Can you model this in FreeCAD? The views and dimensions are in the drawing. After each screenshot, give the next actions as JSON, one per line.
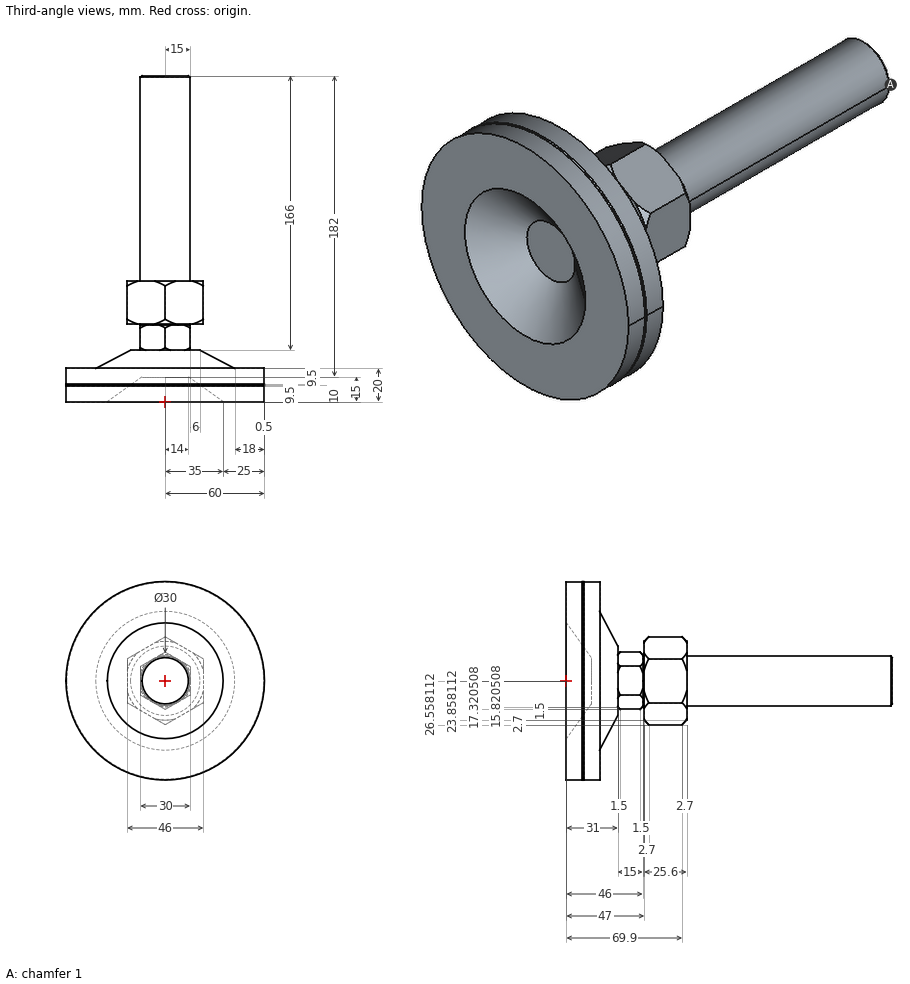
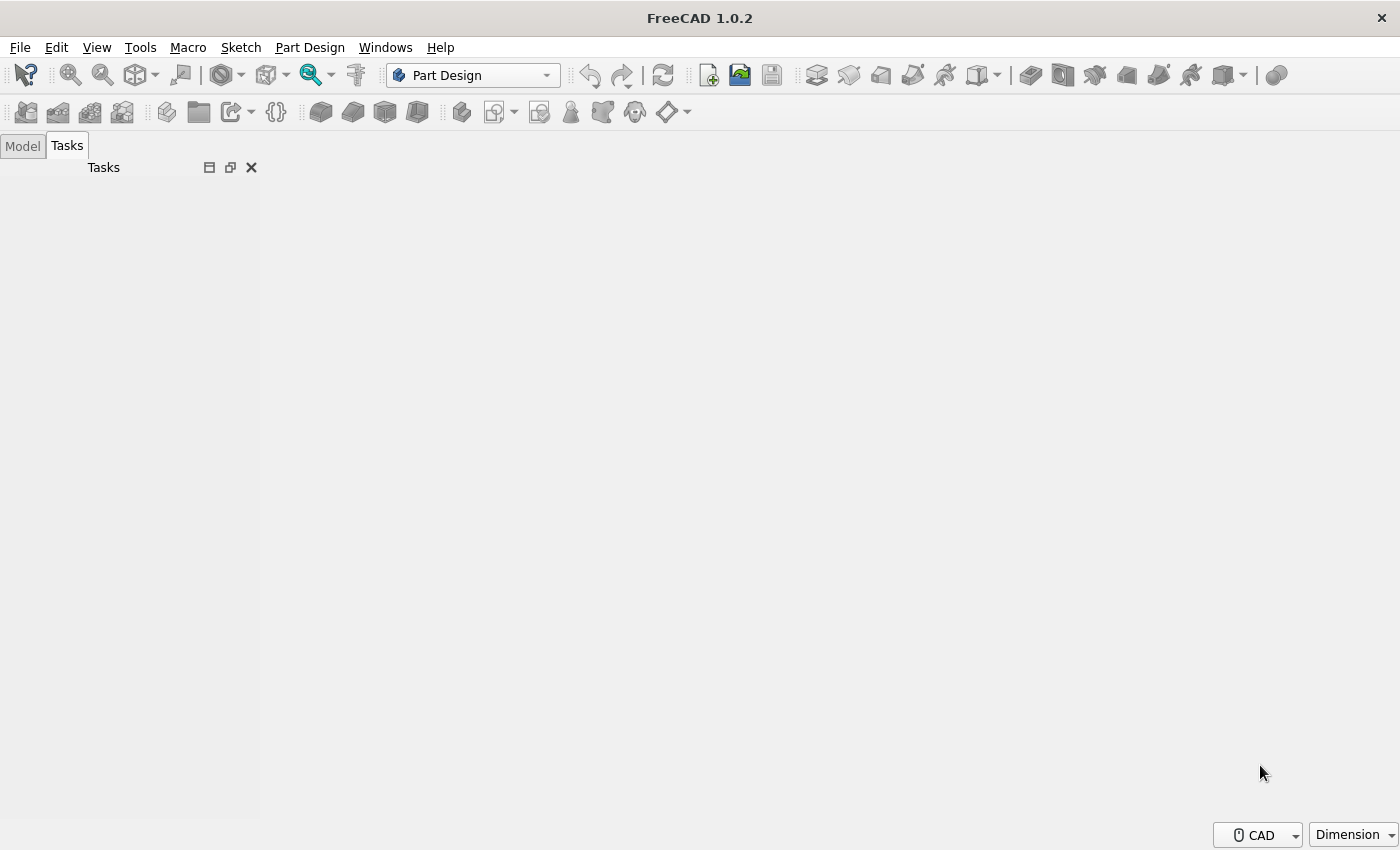
{"action": "key", "text": "ctrl+n"}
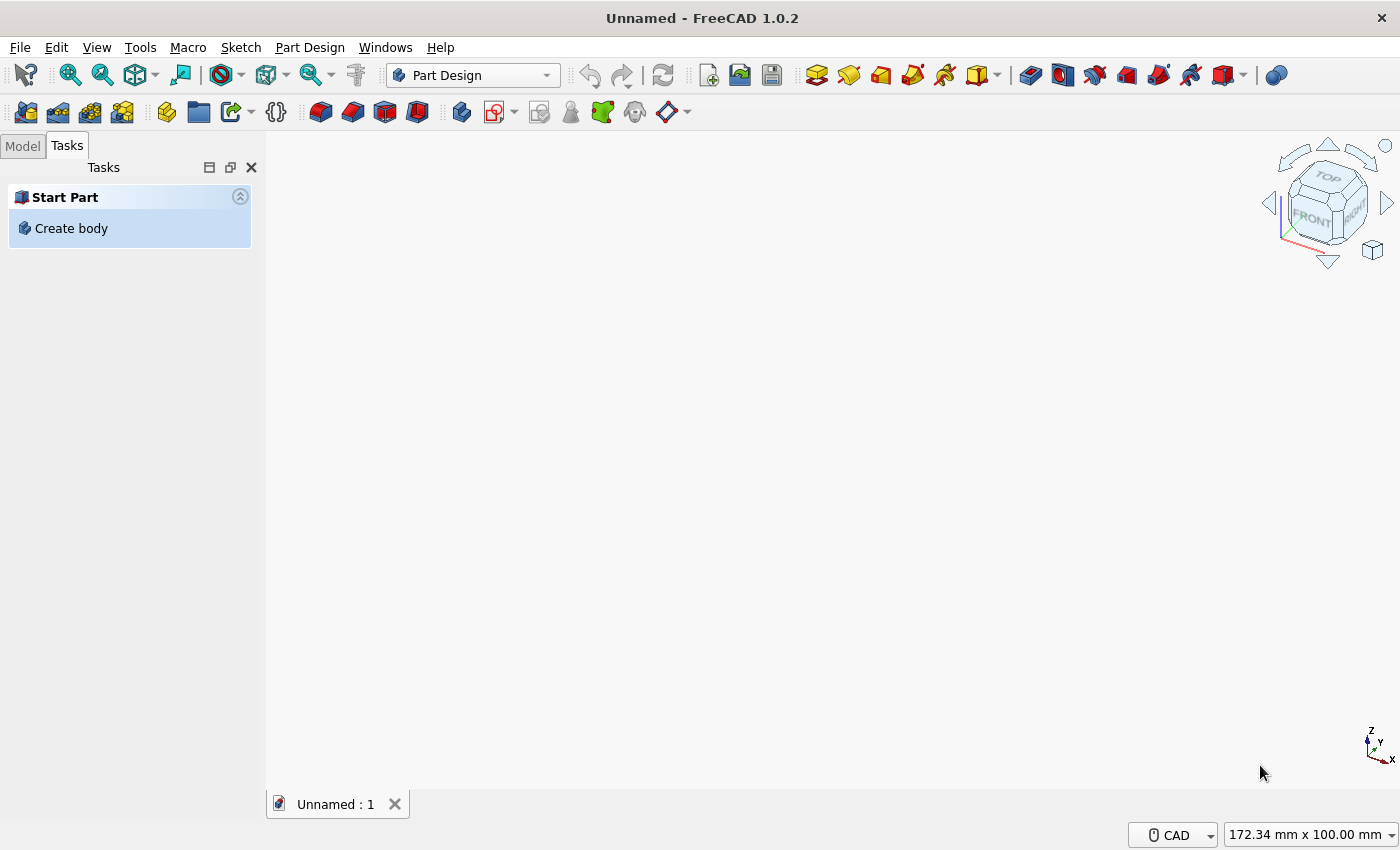
{"action": "left_click", "coordinate": [494, 112]}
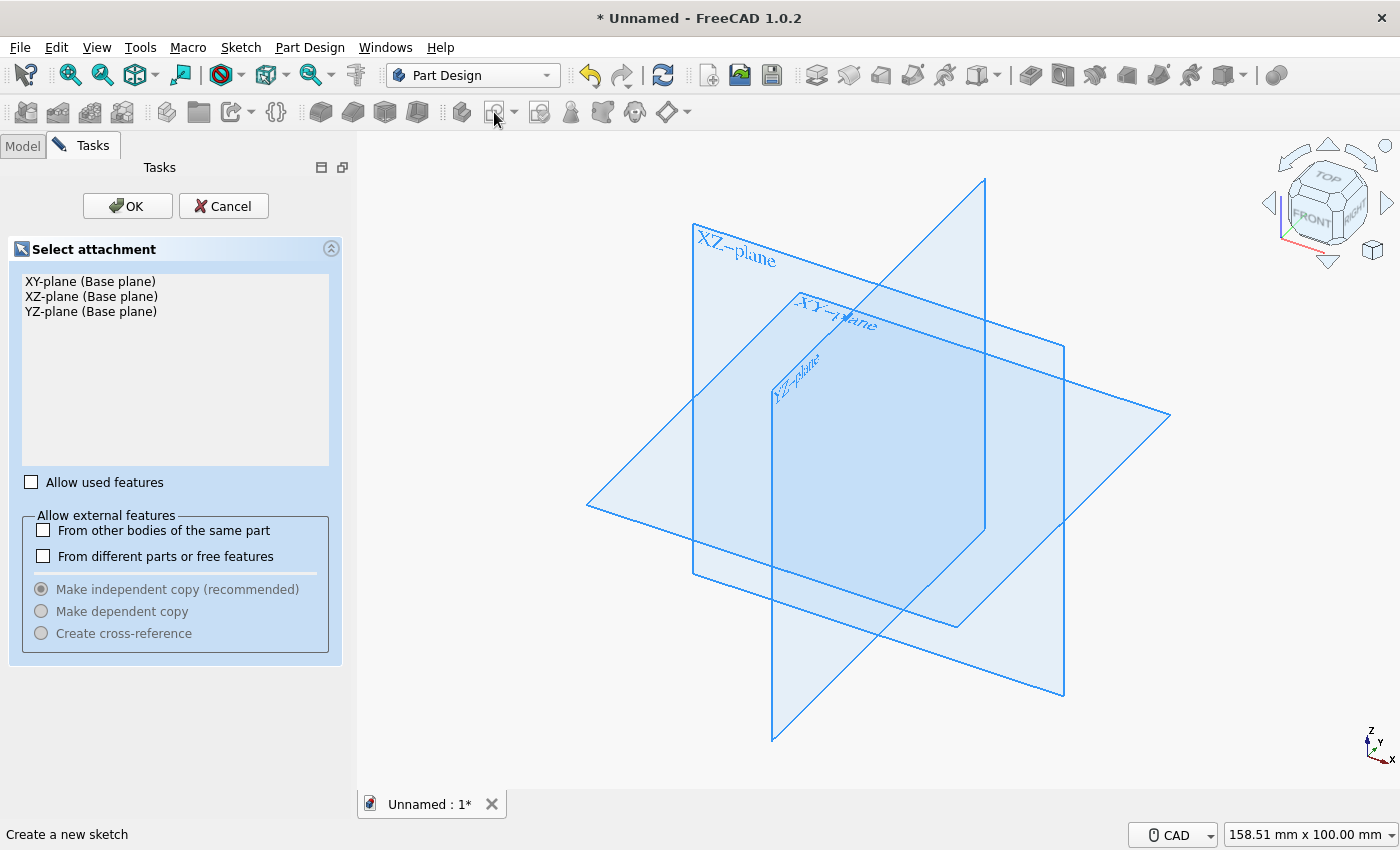
{"action": "left_click", "coordinate": [82, 282]}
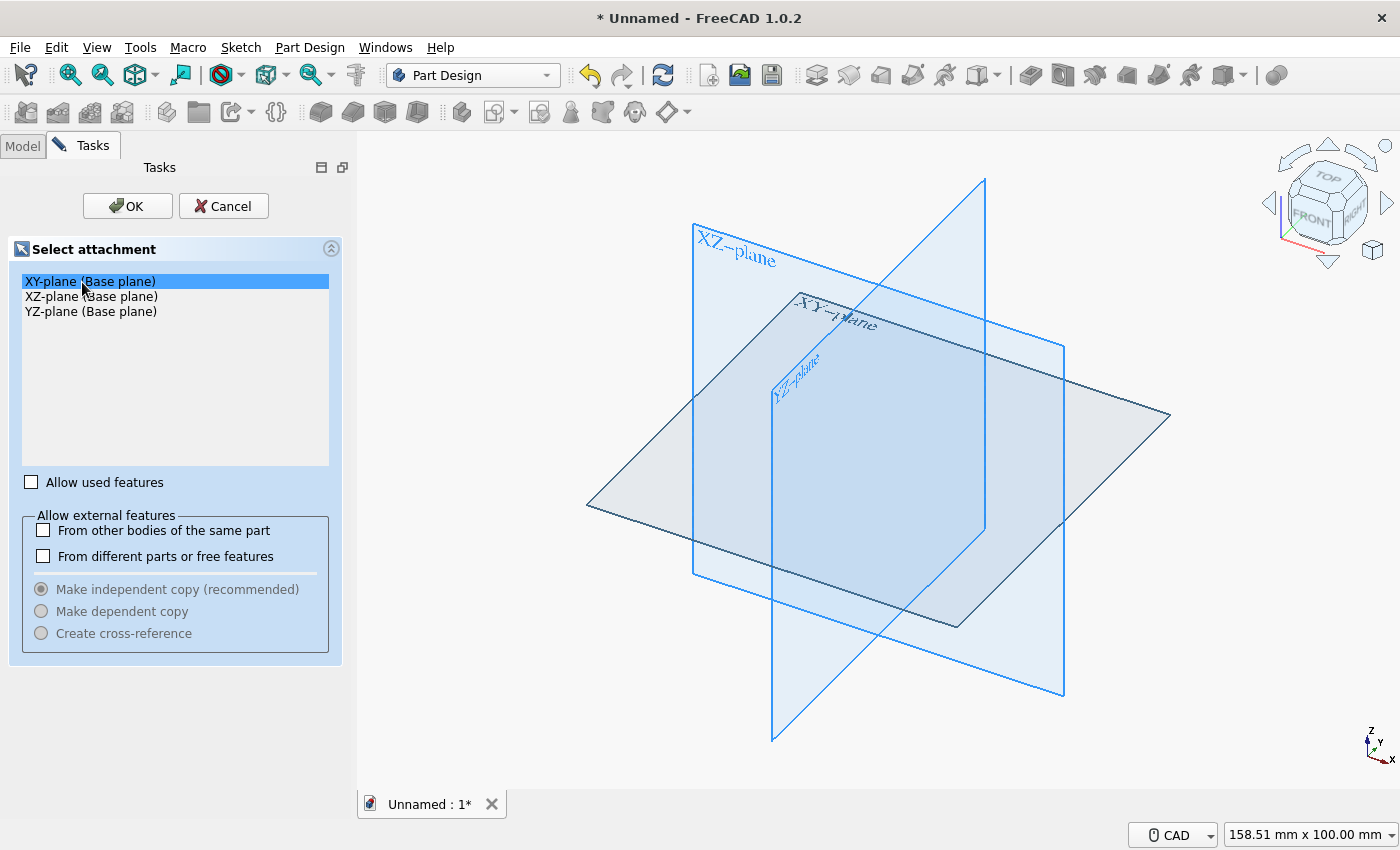
{"action": "left_click", "coordinate": [128, 206]}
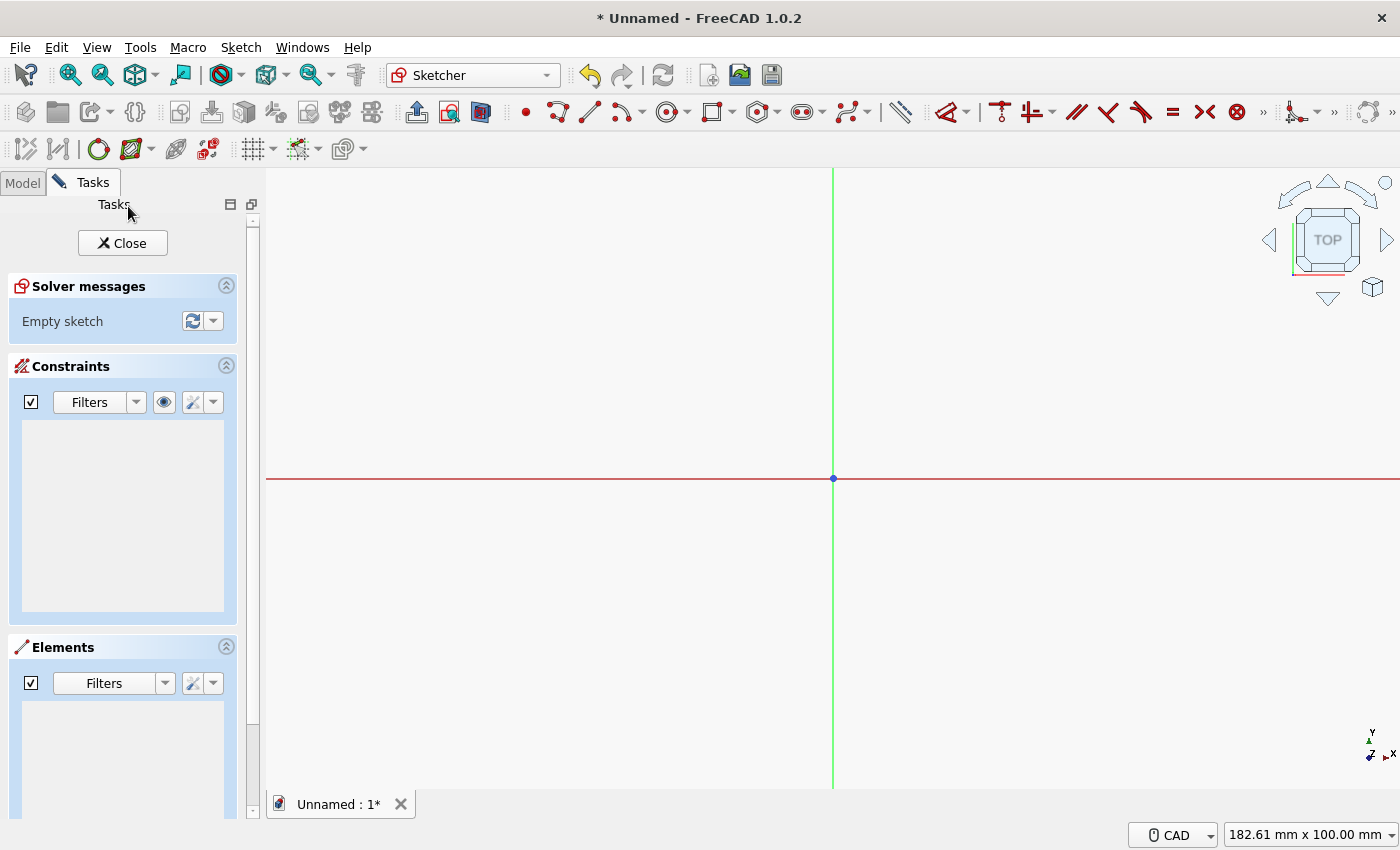
{"action": "scroll", "coordinate": [655, 742], "scroll_direction": "down", "scroll_amount": 6}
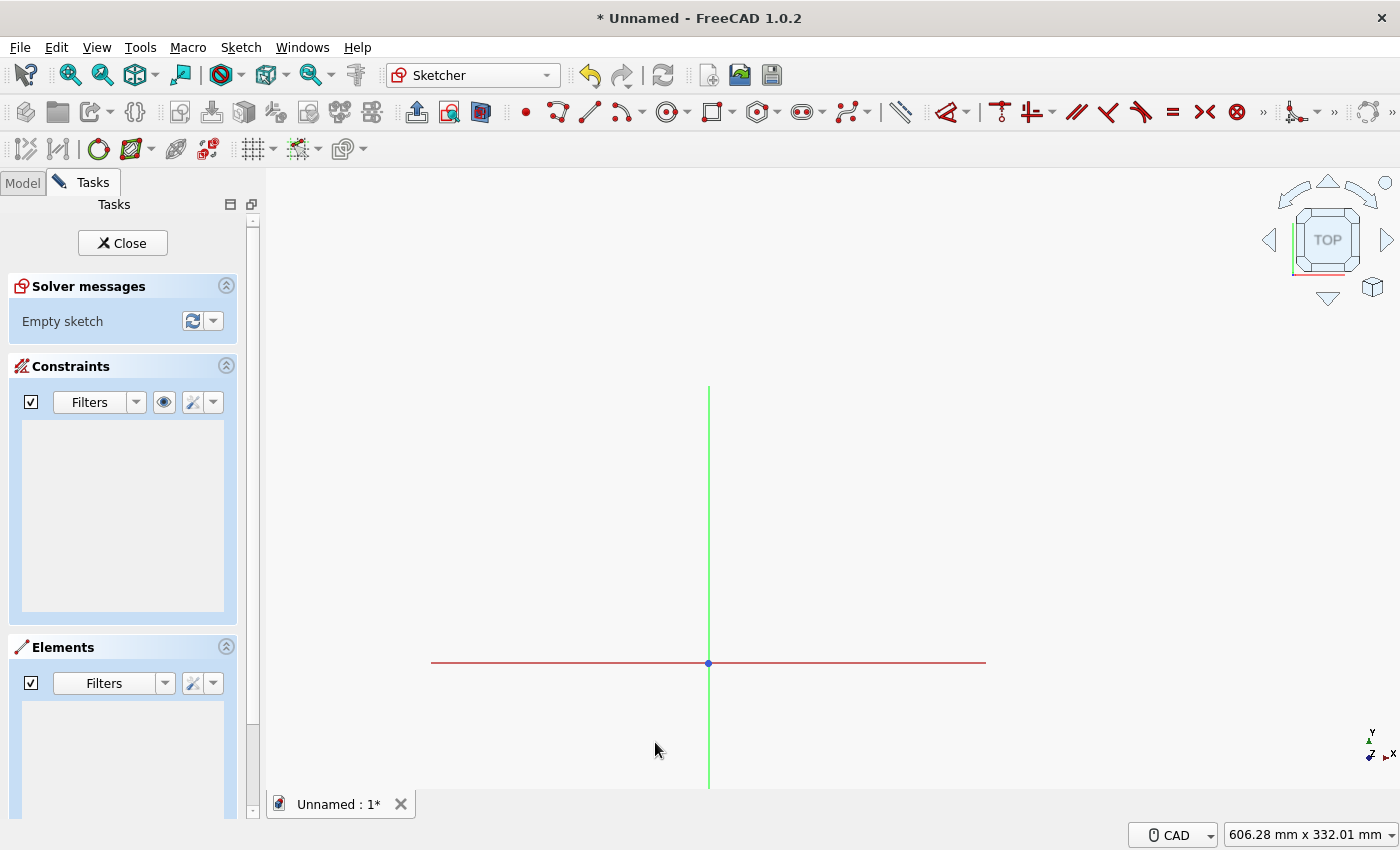
{"action": "left_click", "coordinate": [558, 112]}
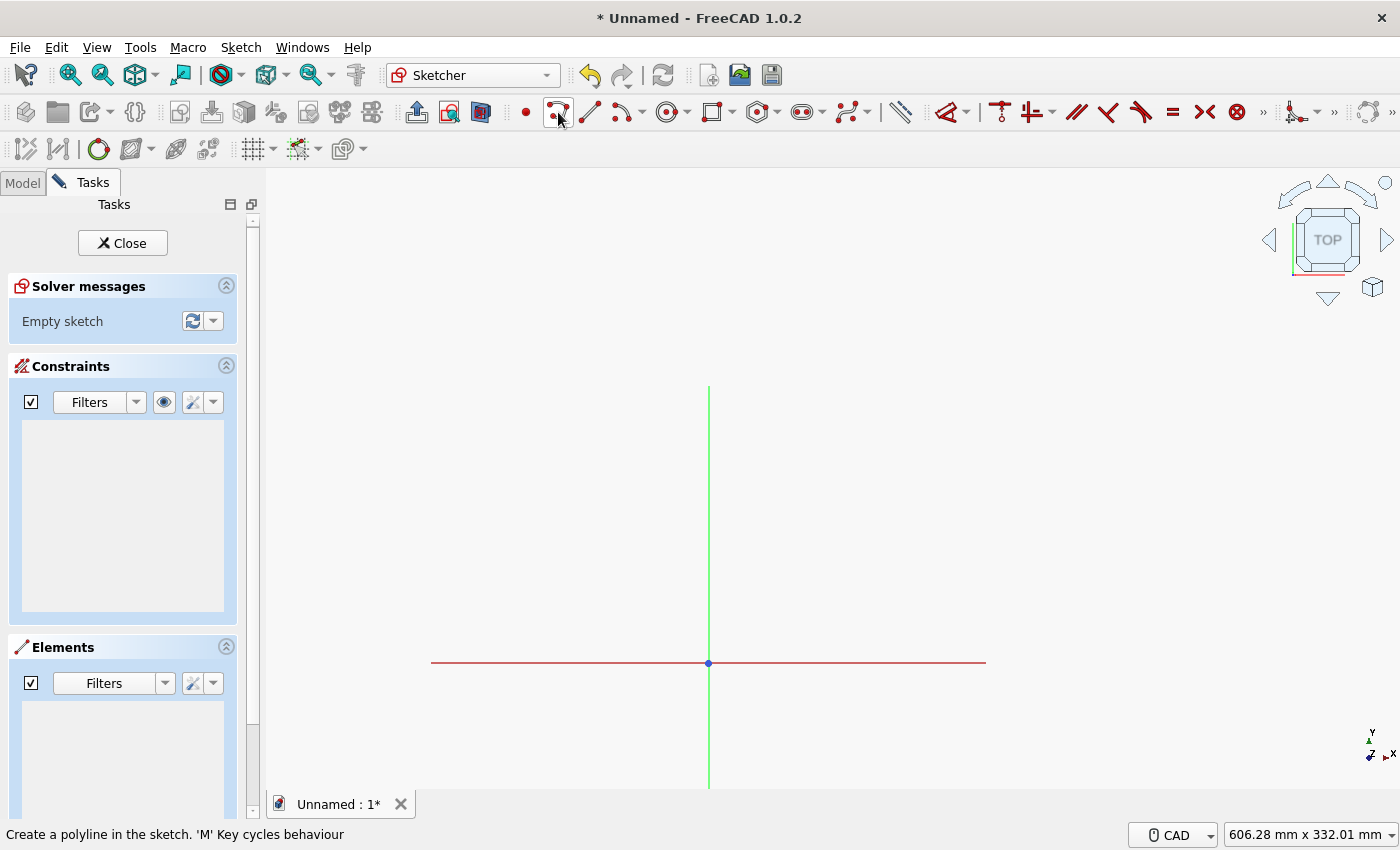
{"action": "left_click", "coordinate": [709, 635]}
{"action": "left_click", "coordinate": [735, 635]}
{"action": "left_click", "coordinate": [774, 663]}
{"action": "left_click", "coordinate": [821, 654]}
{"action": "left_click", "coordinate": [821, 646]}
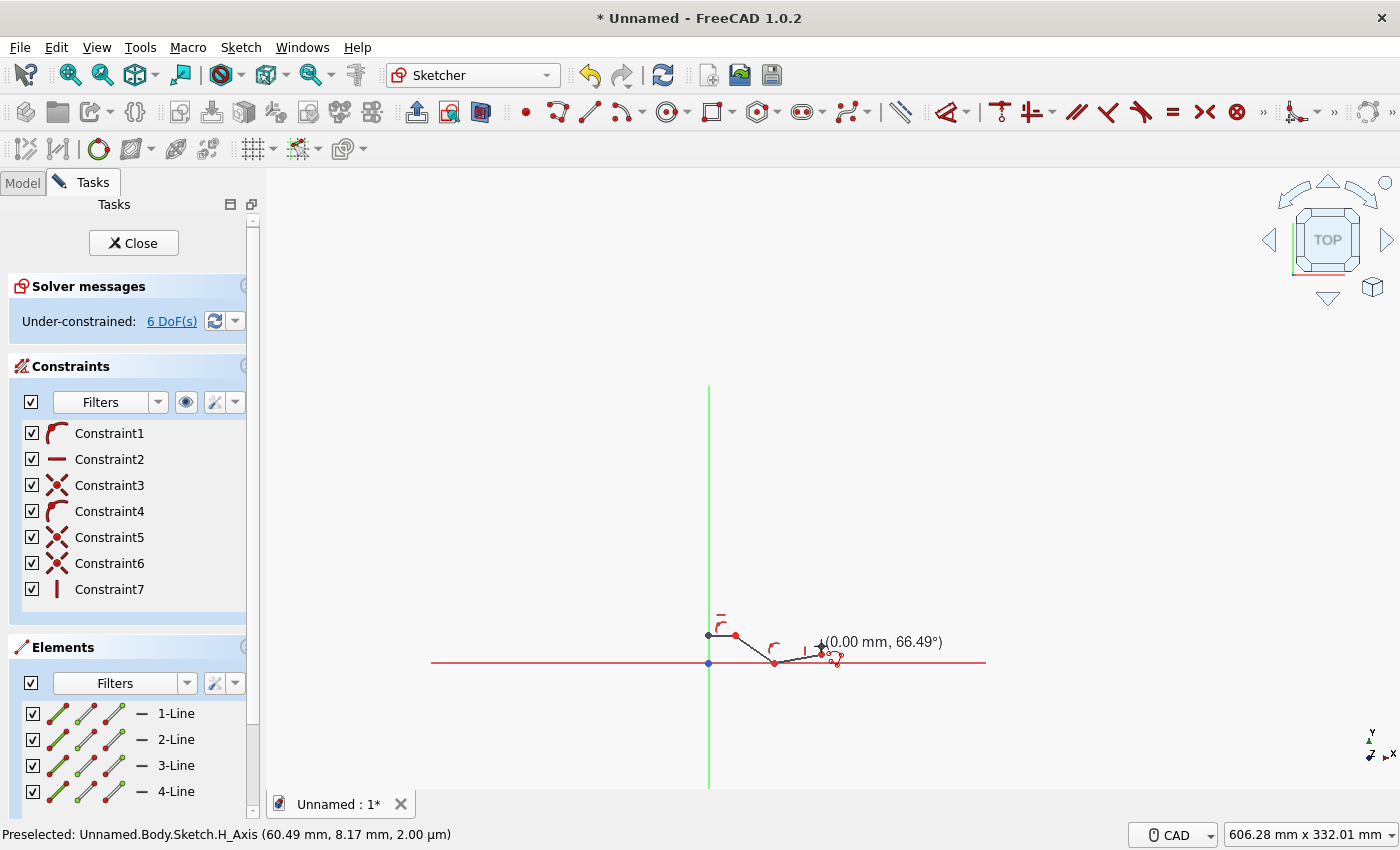
{"action": "scroll", "coordinate": [820, 645], "scroll_direction": "up", "scroll_amount": 13}